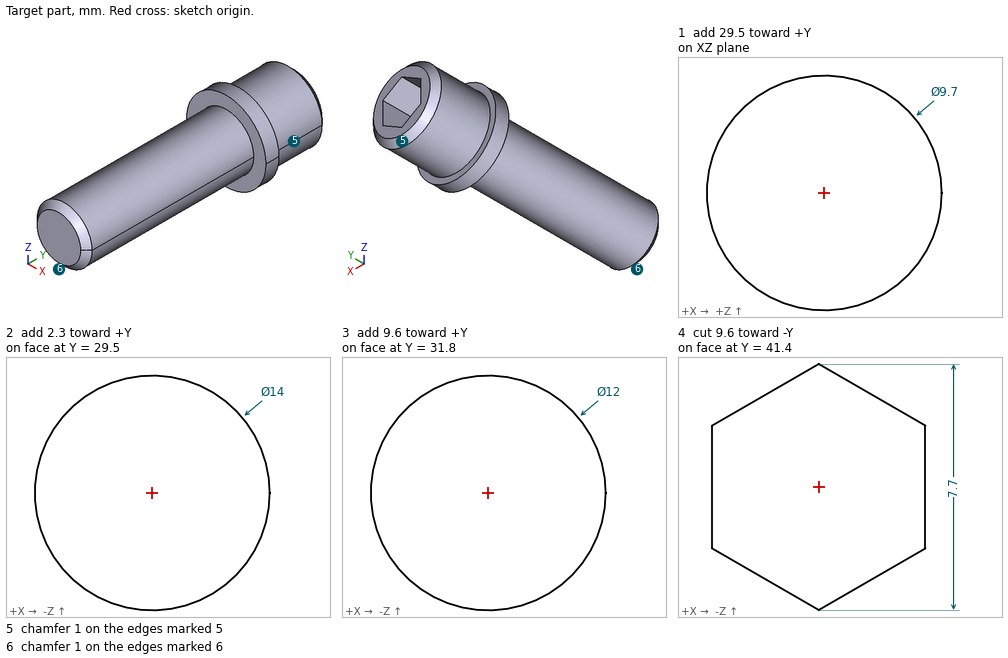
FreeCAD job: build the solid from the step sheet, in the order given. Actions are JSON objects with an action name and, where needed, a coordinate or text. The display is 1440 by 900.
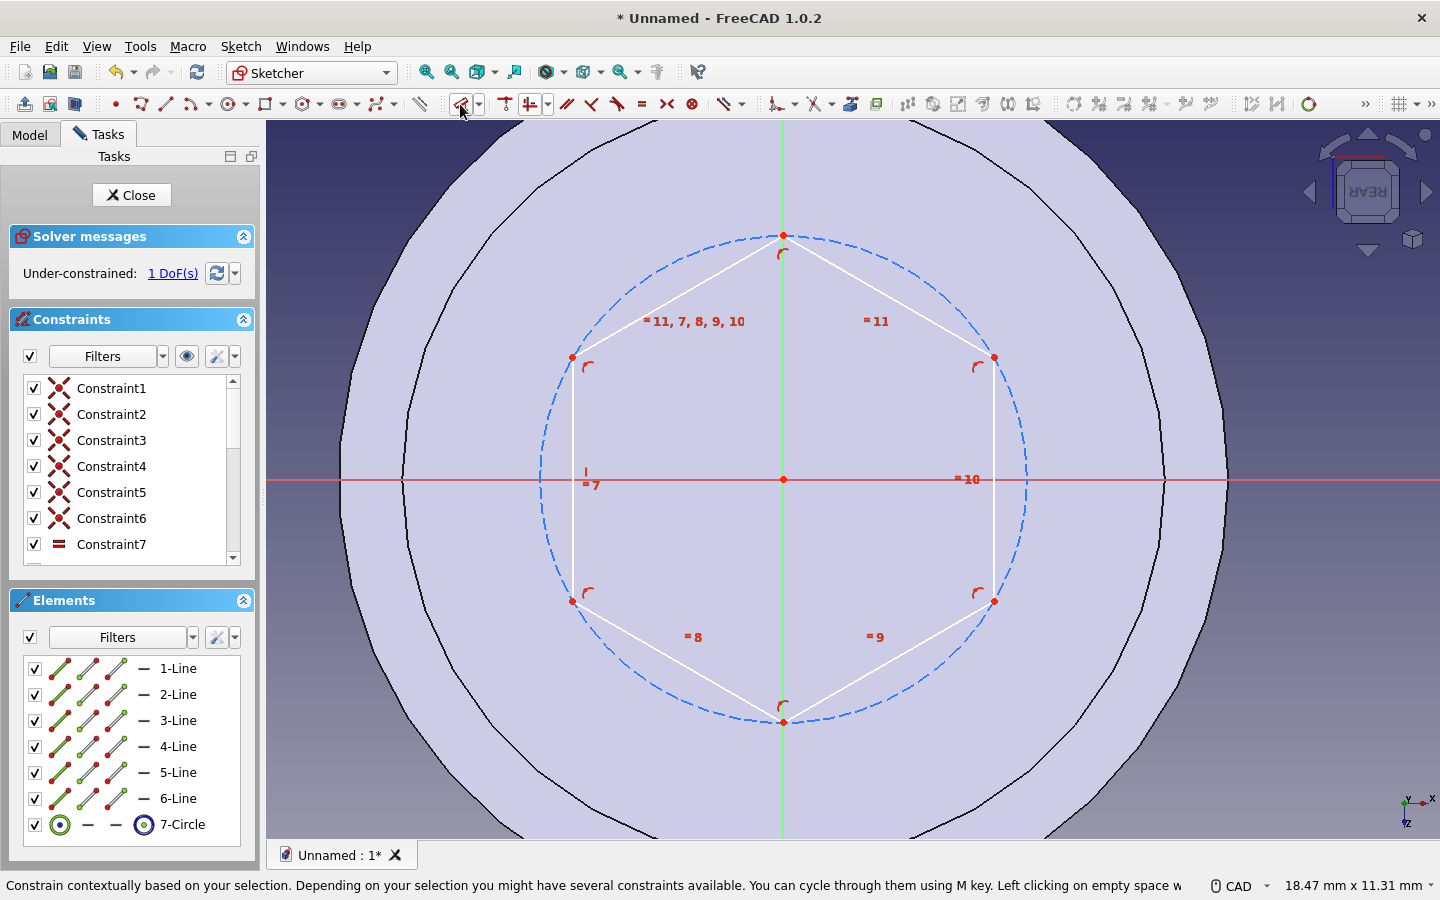
{"action": "left_click", "coordinate": [783, 723]}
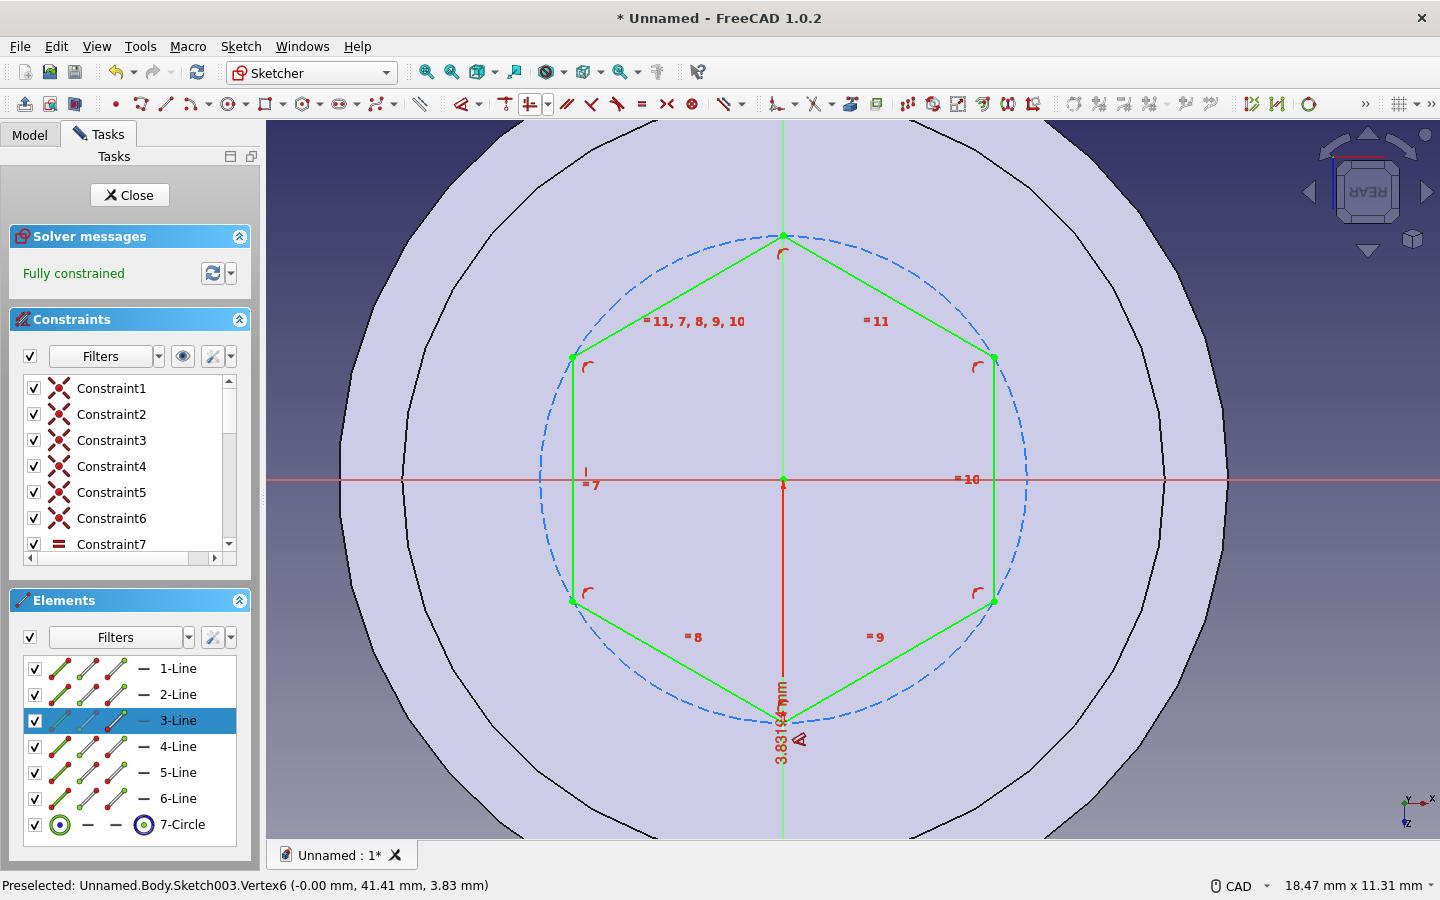
{"action": "left_click", "coordinate": [783, 236]}
{"action": "left_click", "coordinate": [749, 367]}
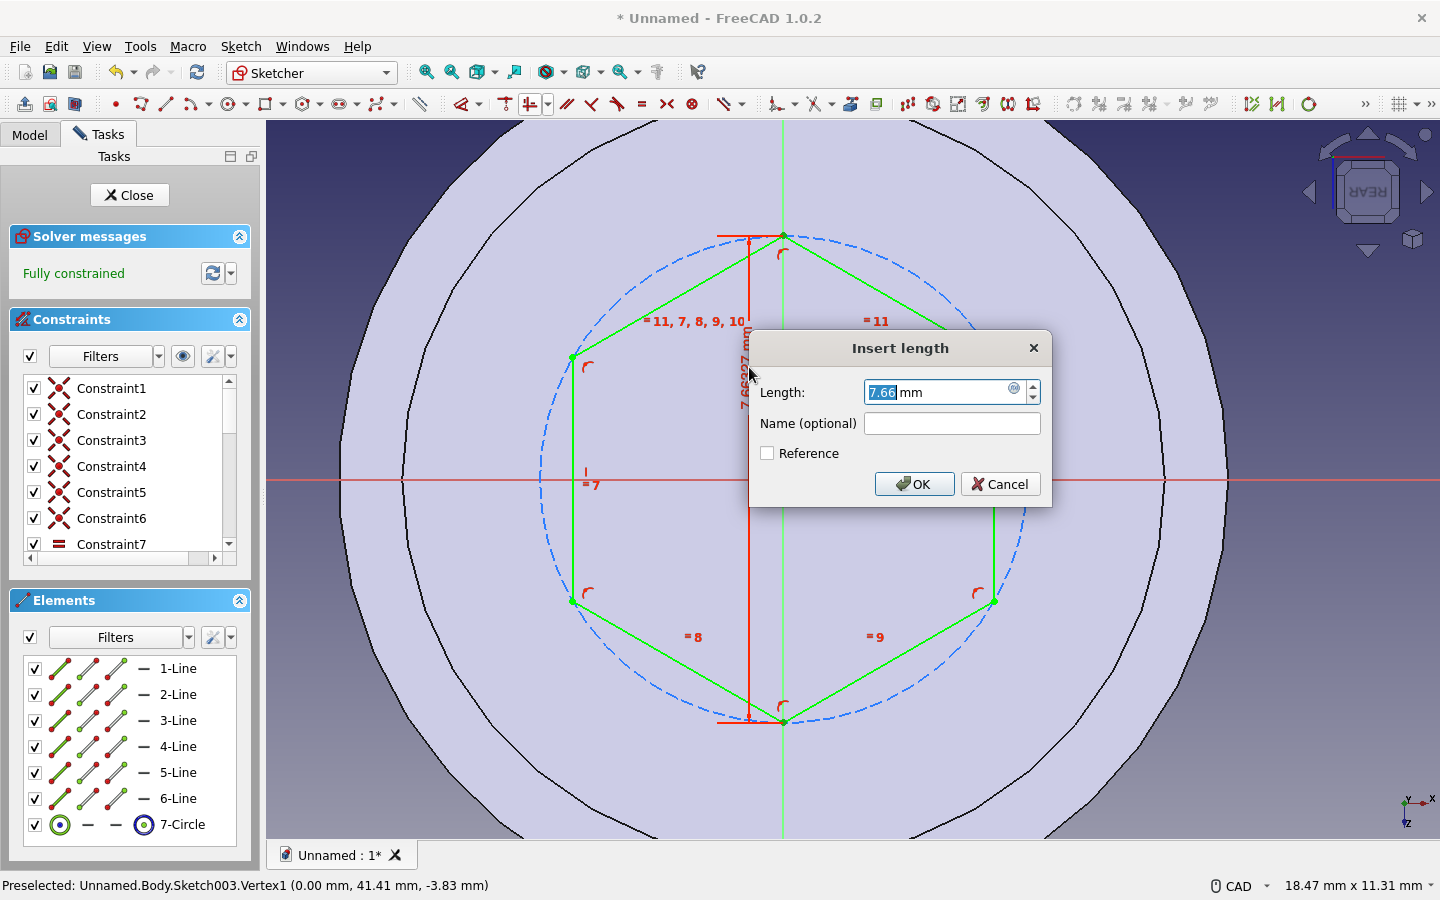
{"action": "type", "text": "7.7"}
{"action": "key", "text": "Return"}
{"action": "key", "text": "Escape"}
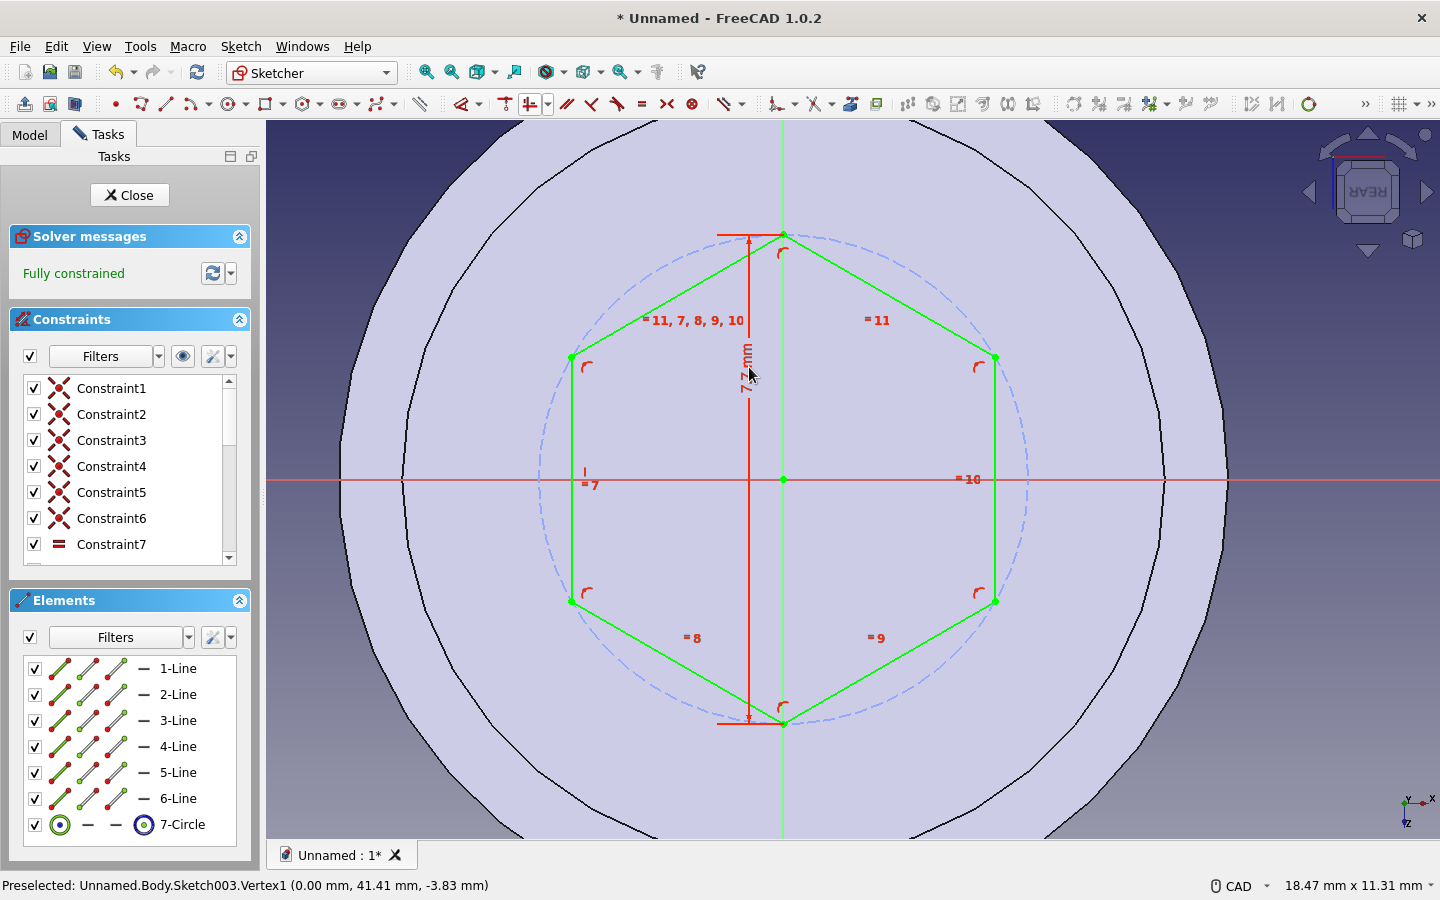
{"action": "left_click", "coordinate": [130, 195]}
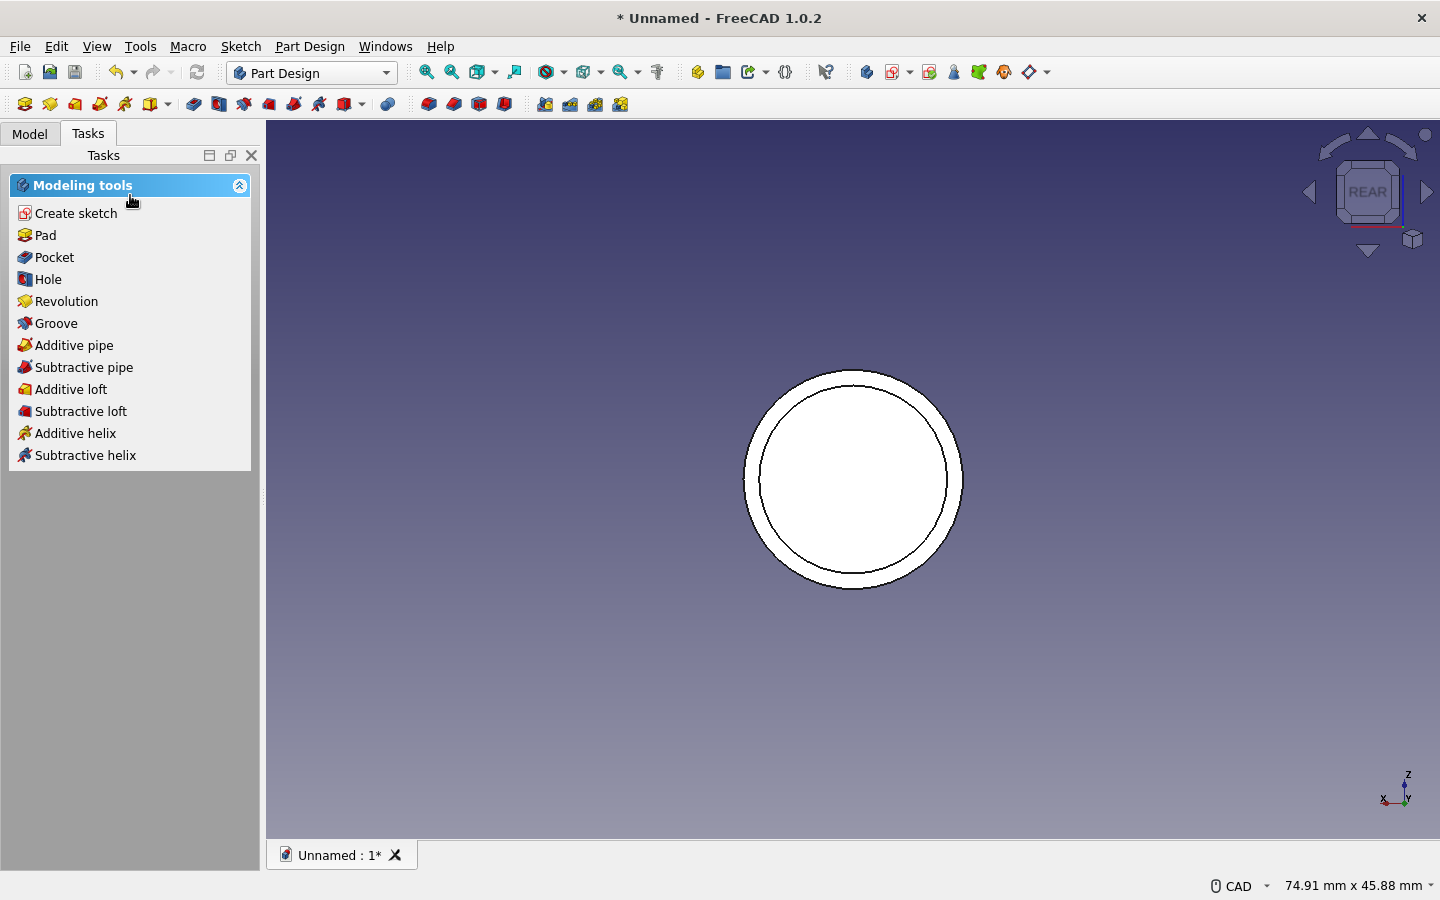
{"action": "left_click", "coordinate": [194, 104]}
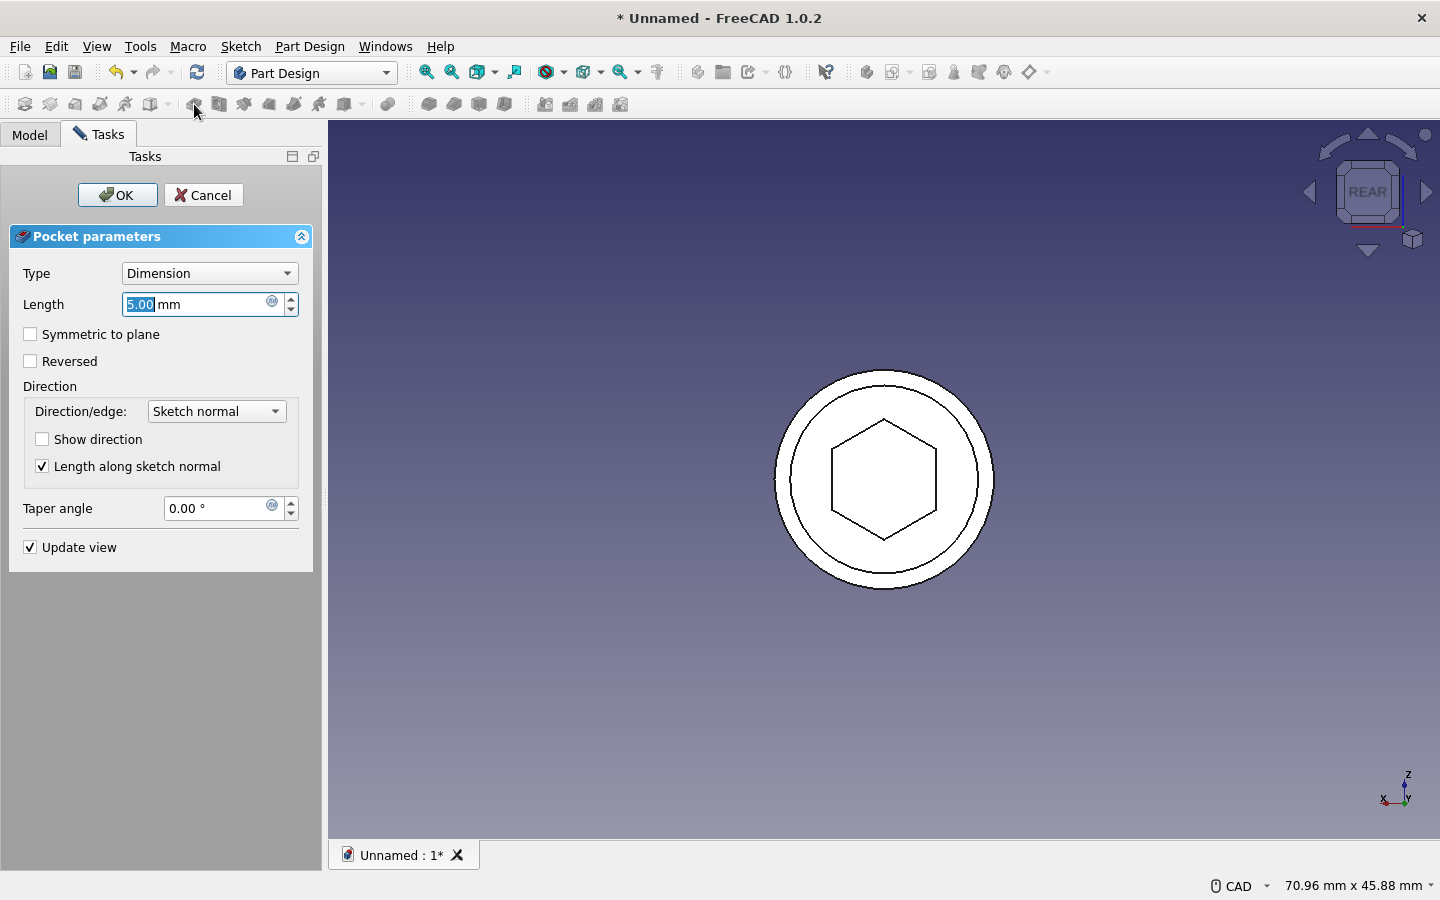
{"action": "type", "text": "9.6"}
{"action": "key", "text": "Tab"}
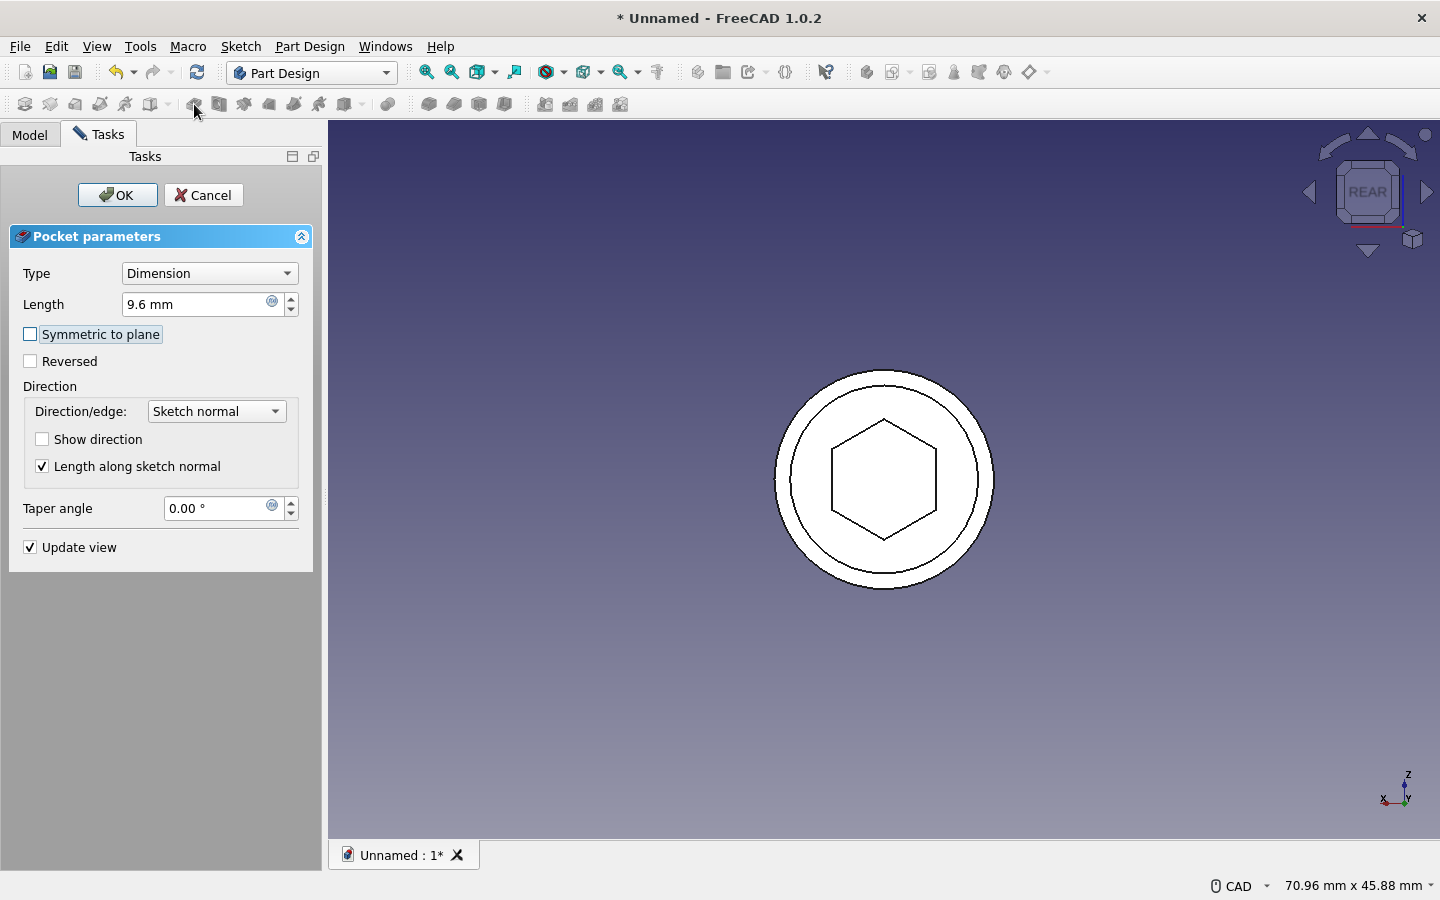
{"action": "left_click", "coordinate": [118, 195]}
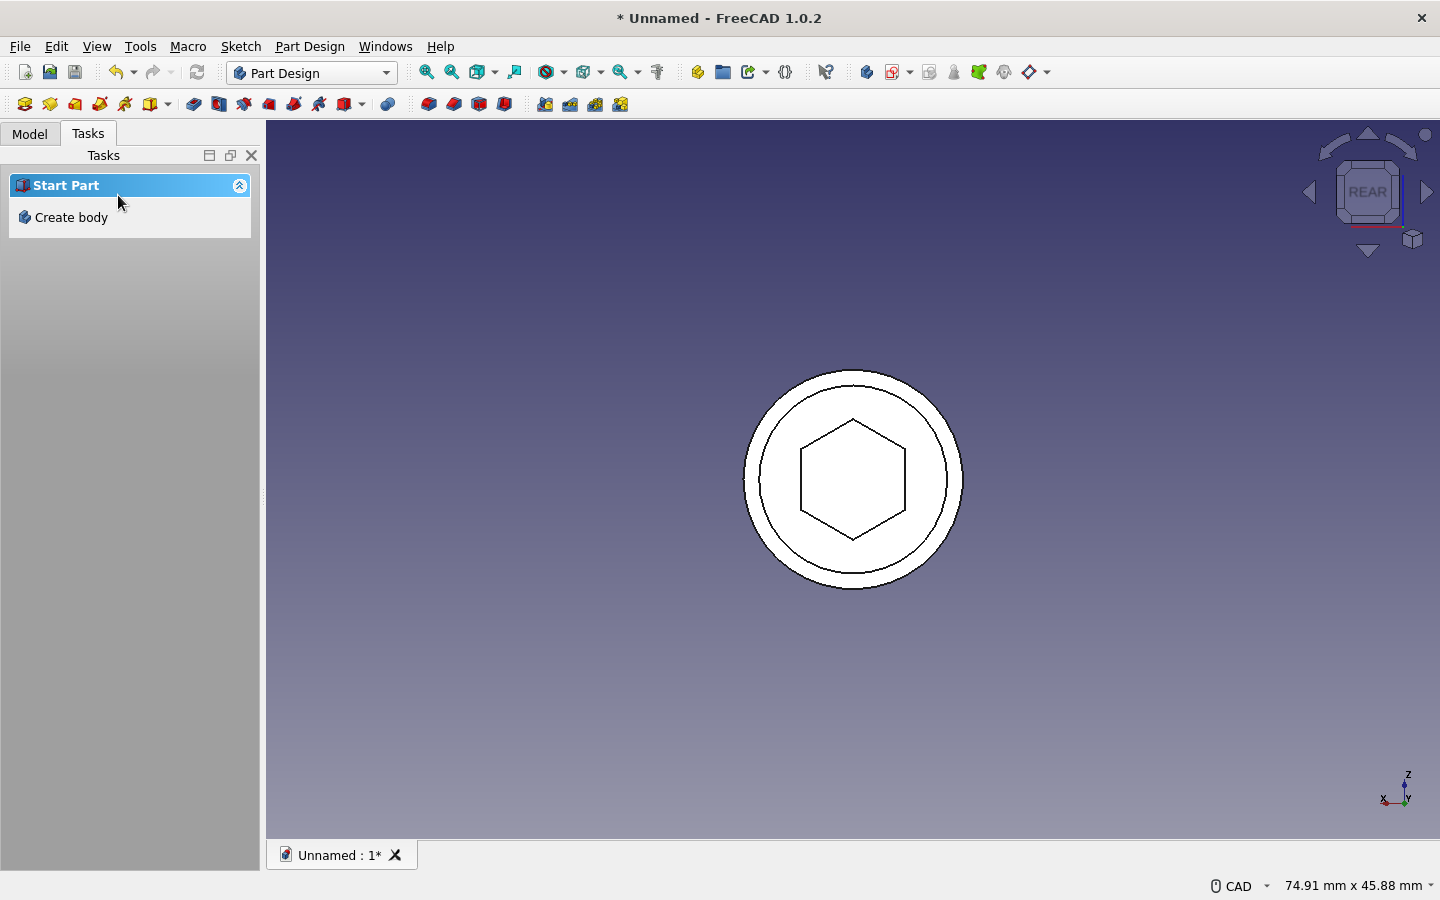
{"action": "left_click", "coordinate": [427, 72]}